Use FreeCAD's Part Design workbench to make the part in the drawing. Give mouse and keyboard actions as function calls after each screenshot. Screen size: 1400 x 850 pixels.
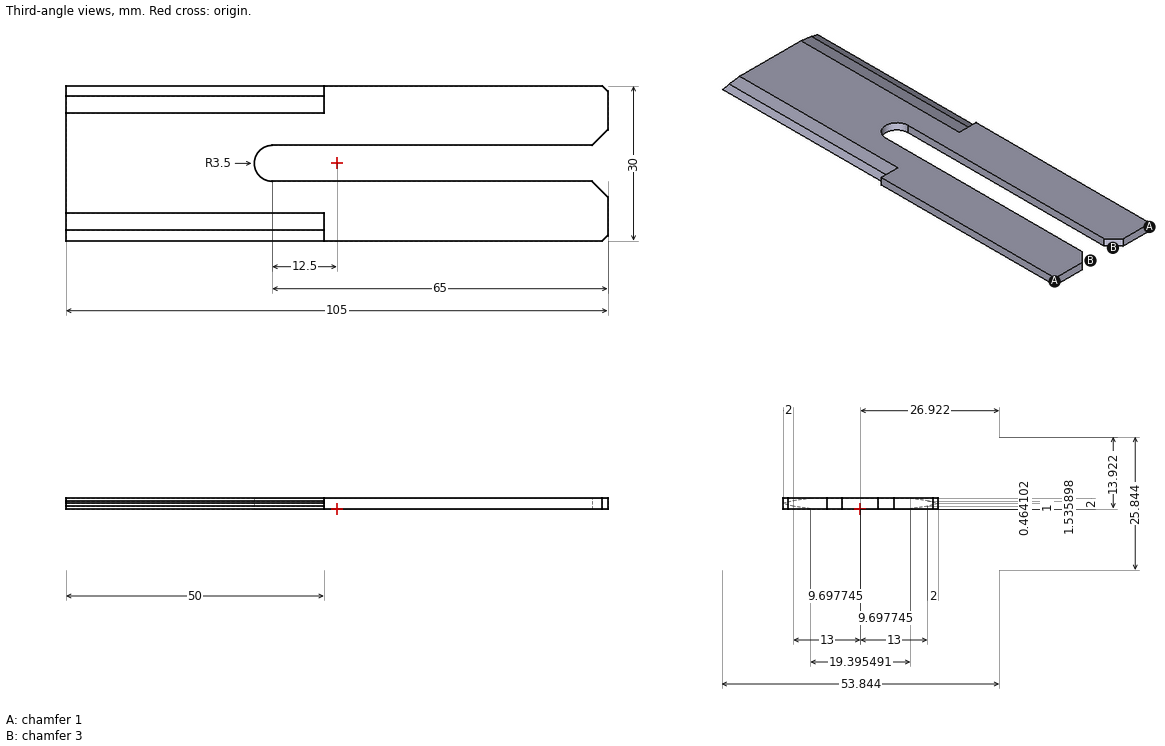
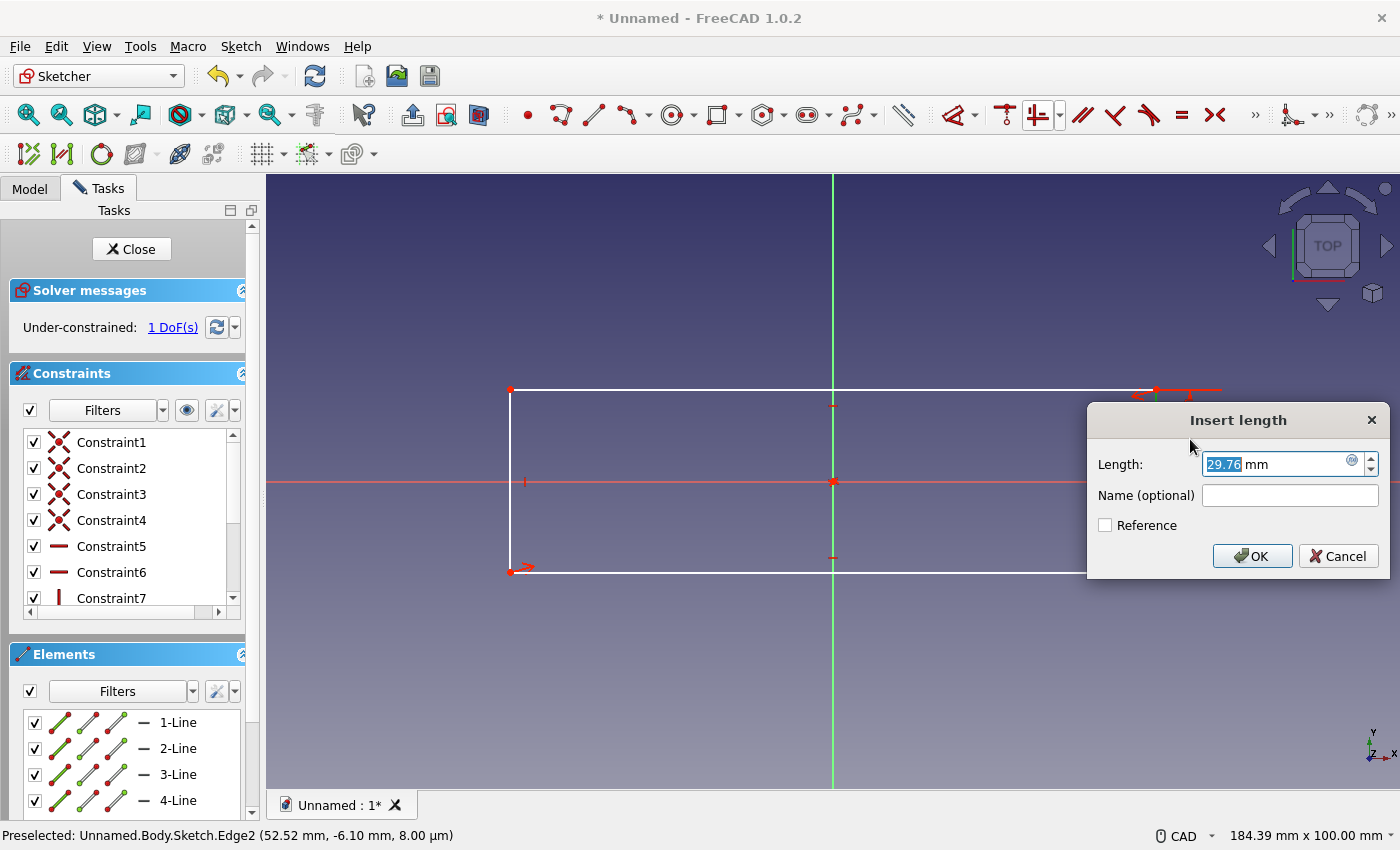
text(30)
key(Return)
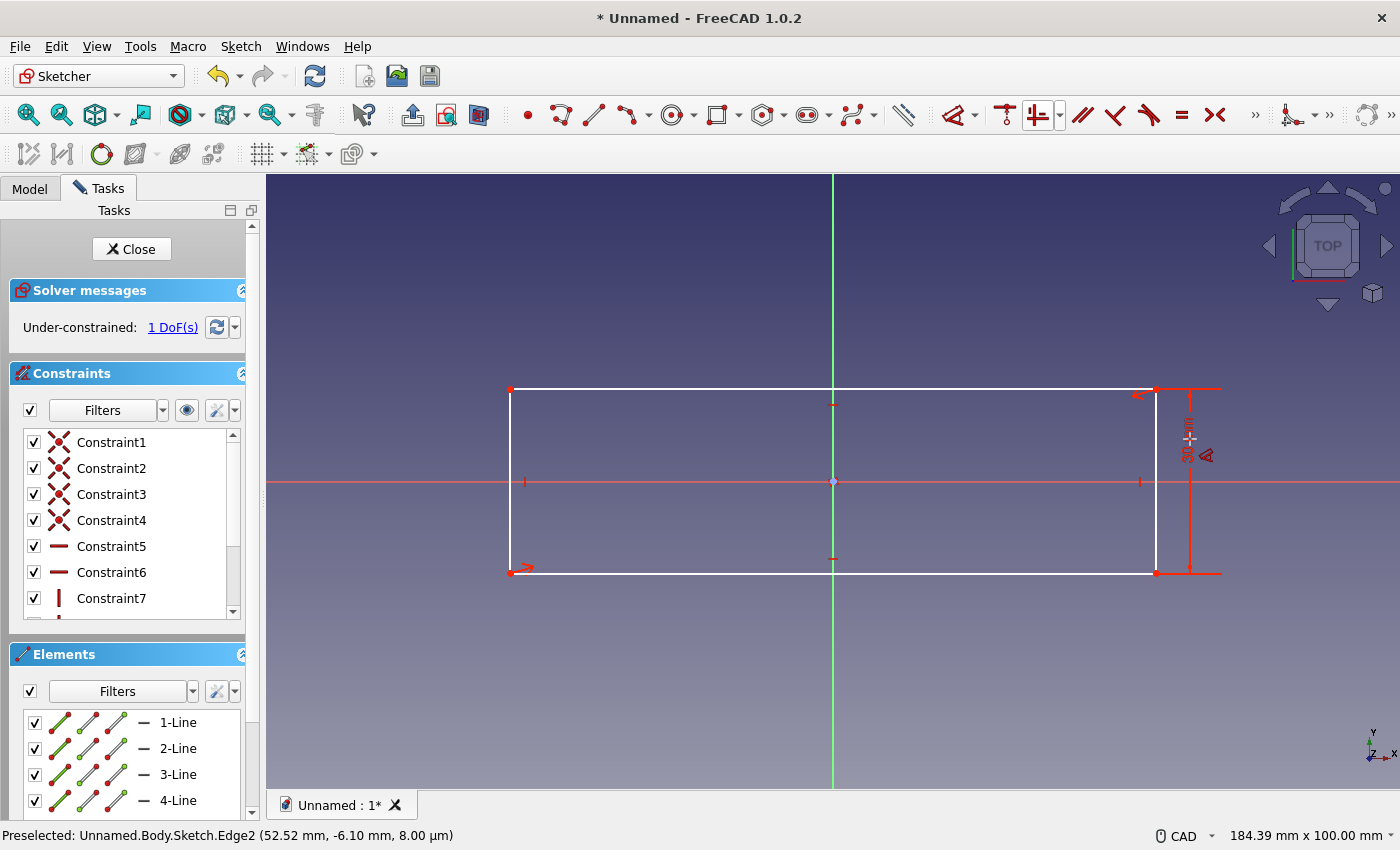
click(704, 574)
click(684, 608)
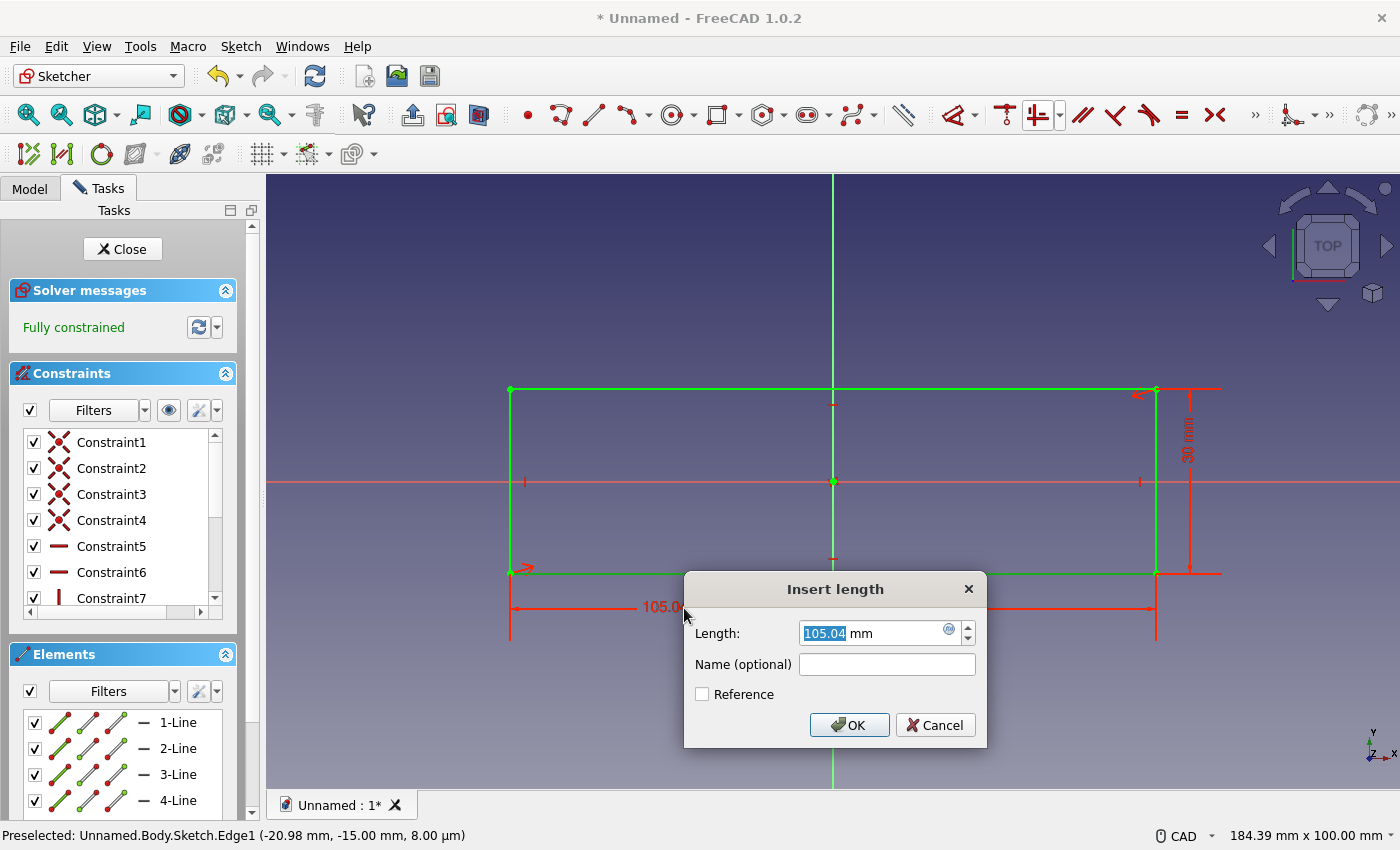
text(105)
key(Return)
key(Escape)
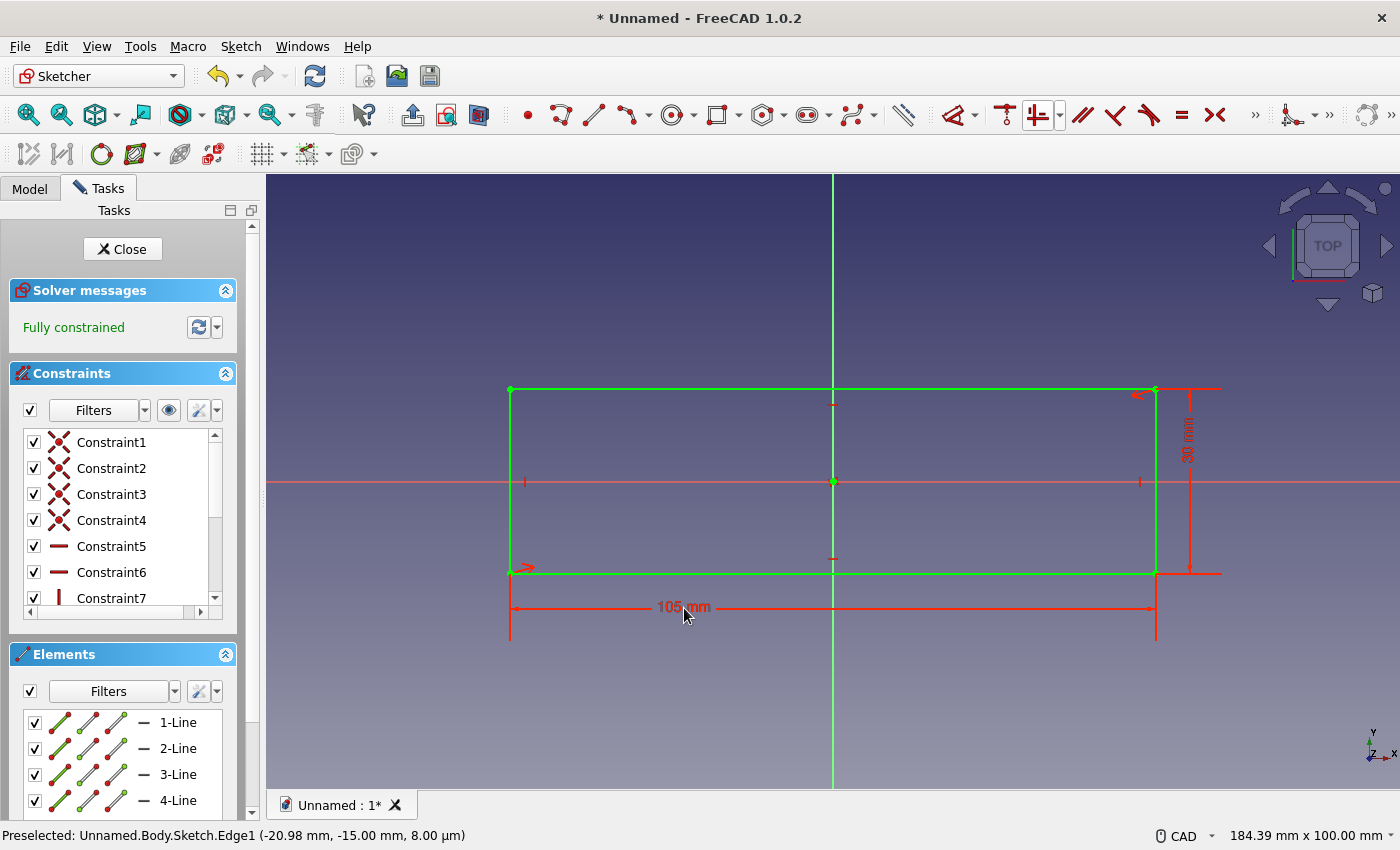
click(123, 249)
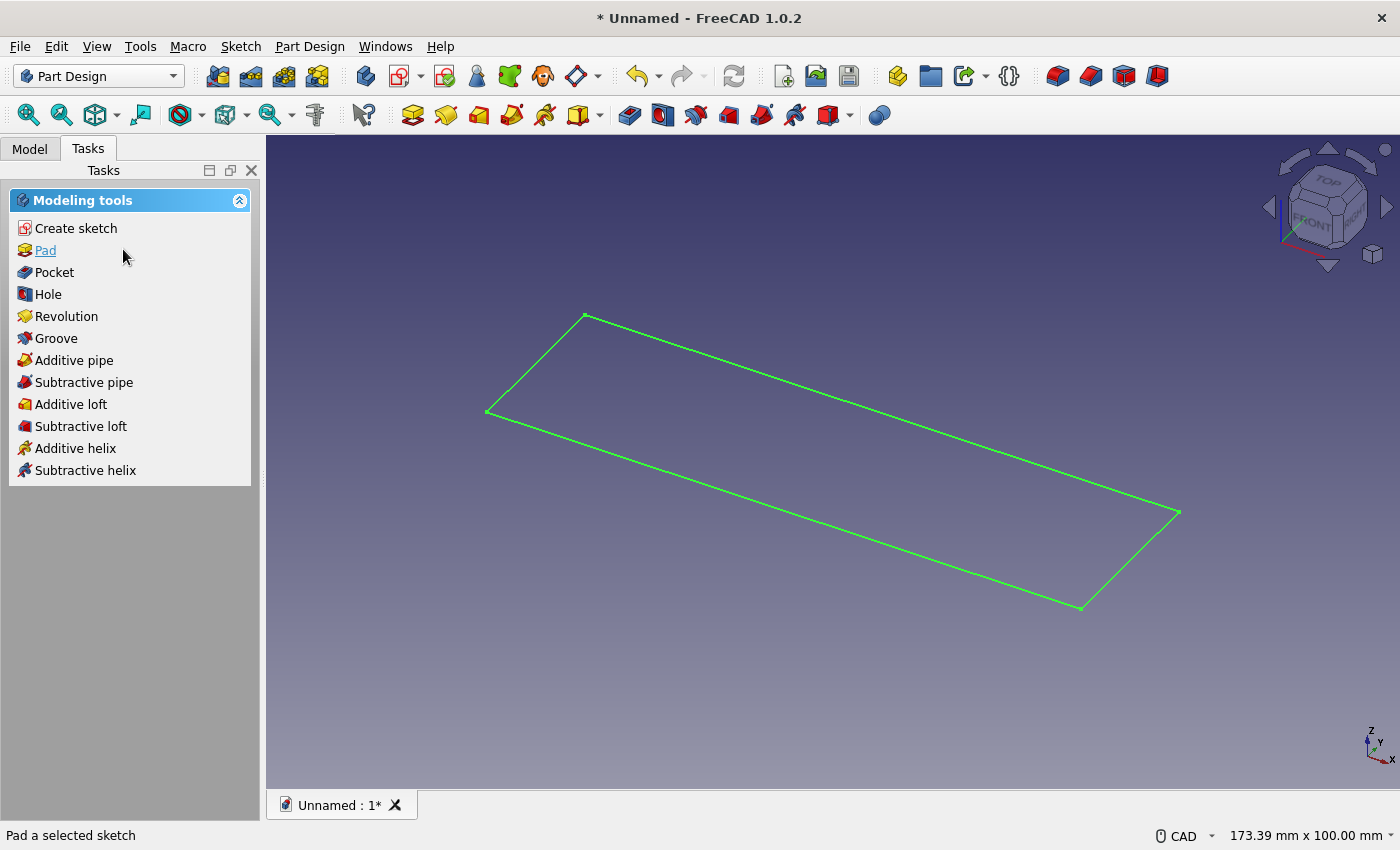
click(413, 116)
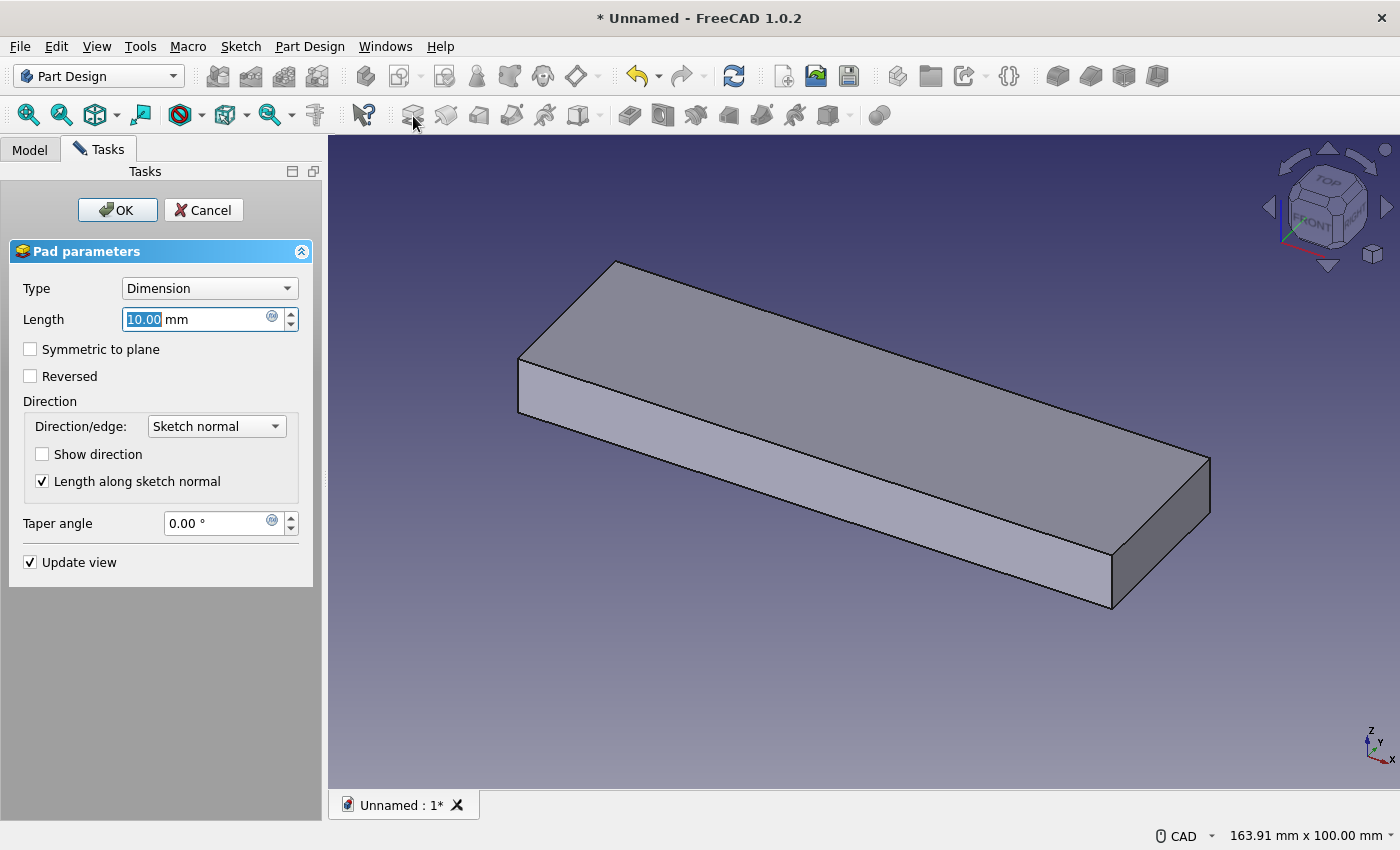
text(2)
key(Tab)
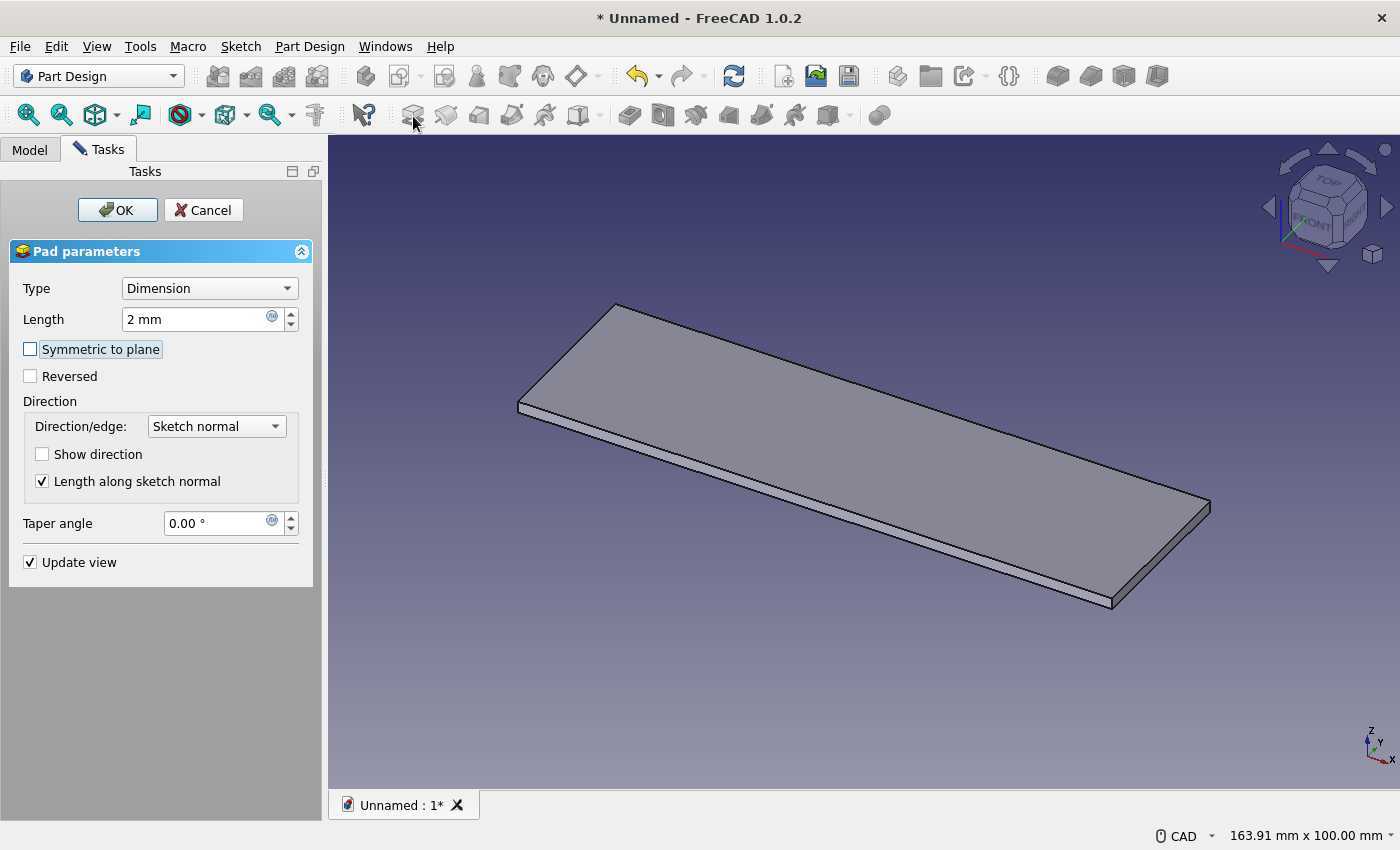
click(118, 210)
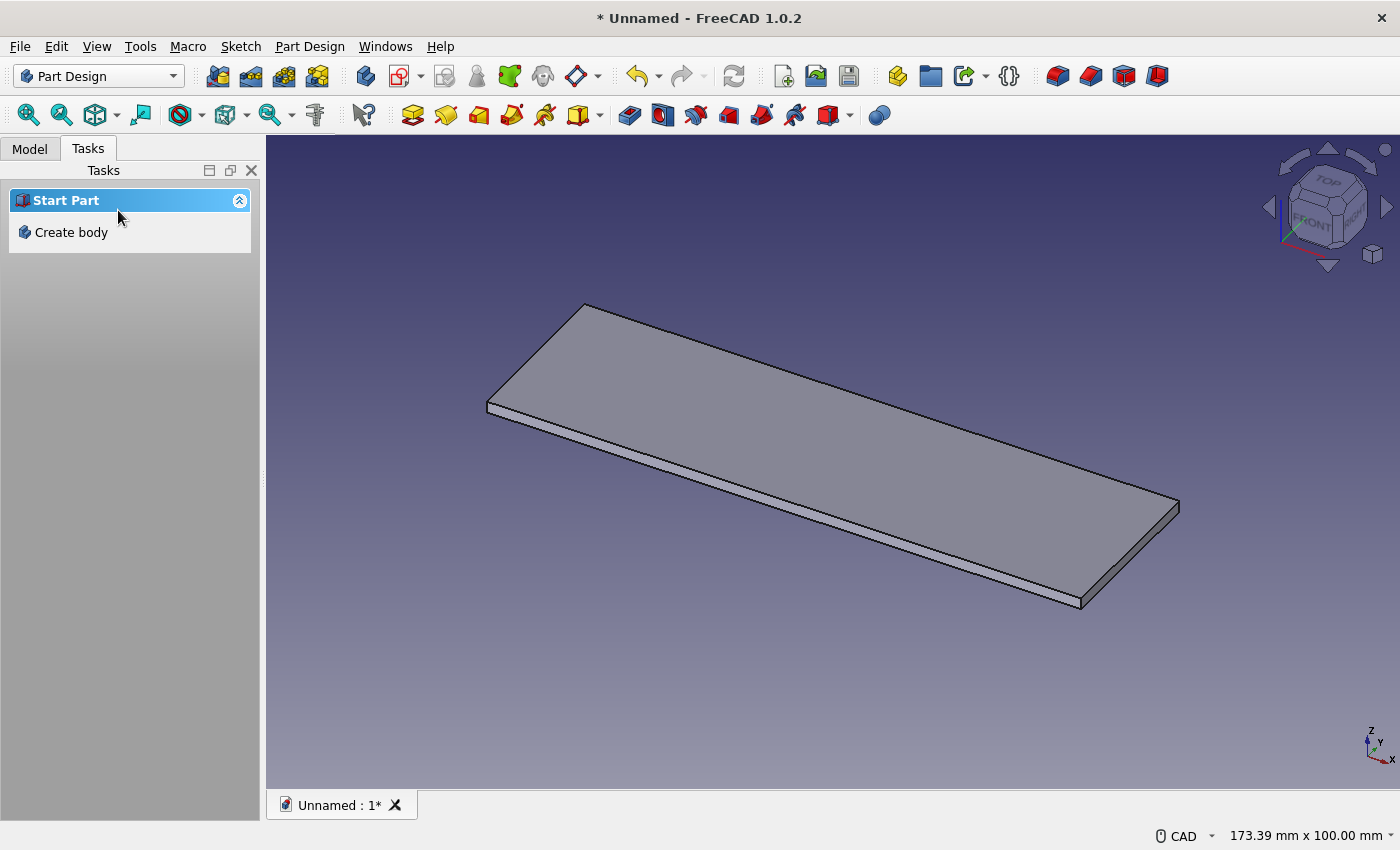
click(1003, 507)